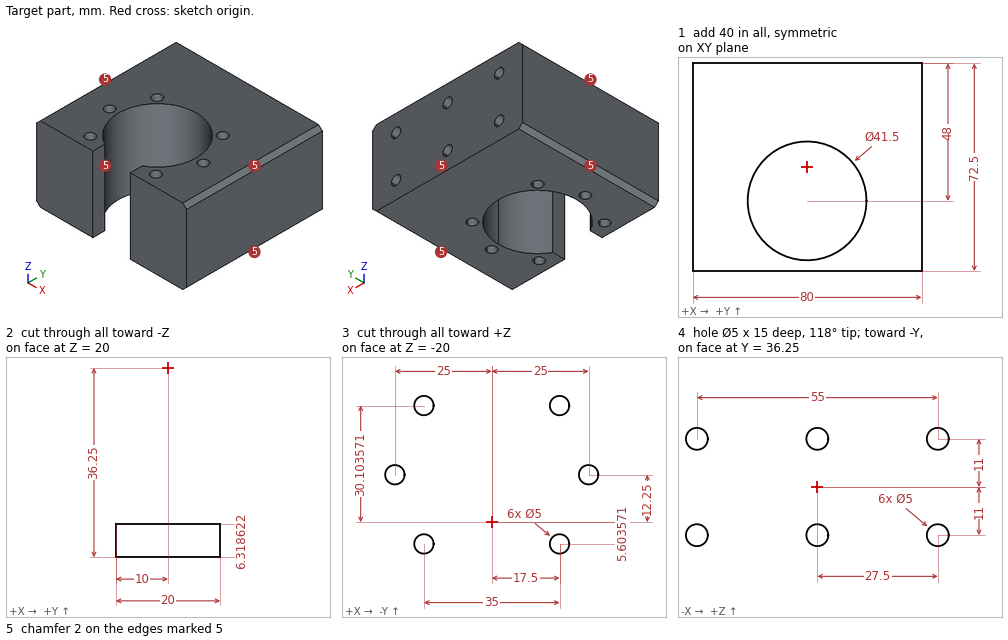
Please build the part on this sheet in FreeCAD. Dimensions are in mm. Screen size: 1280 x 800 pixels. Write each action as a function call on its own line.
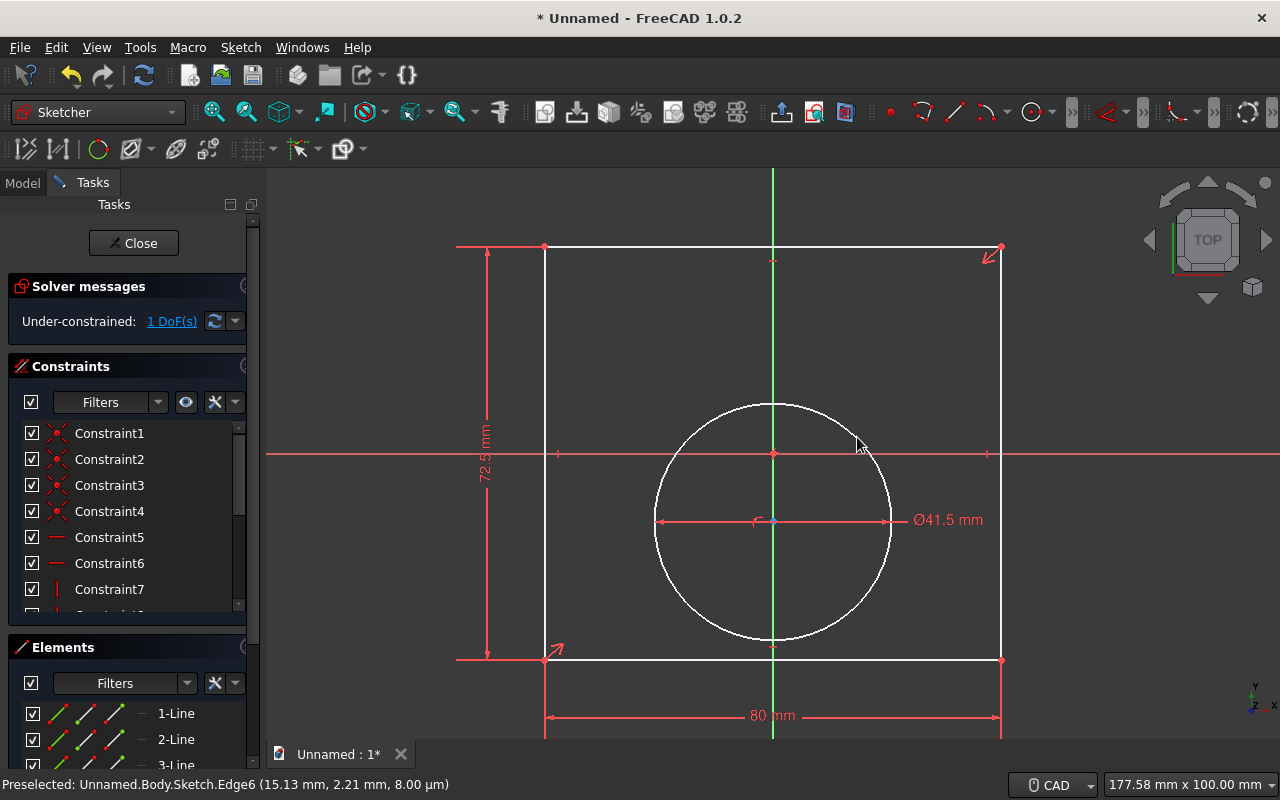
click(1106, 112)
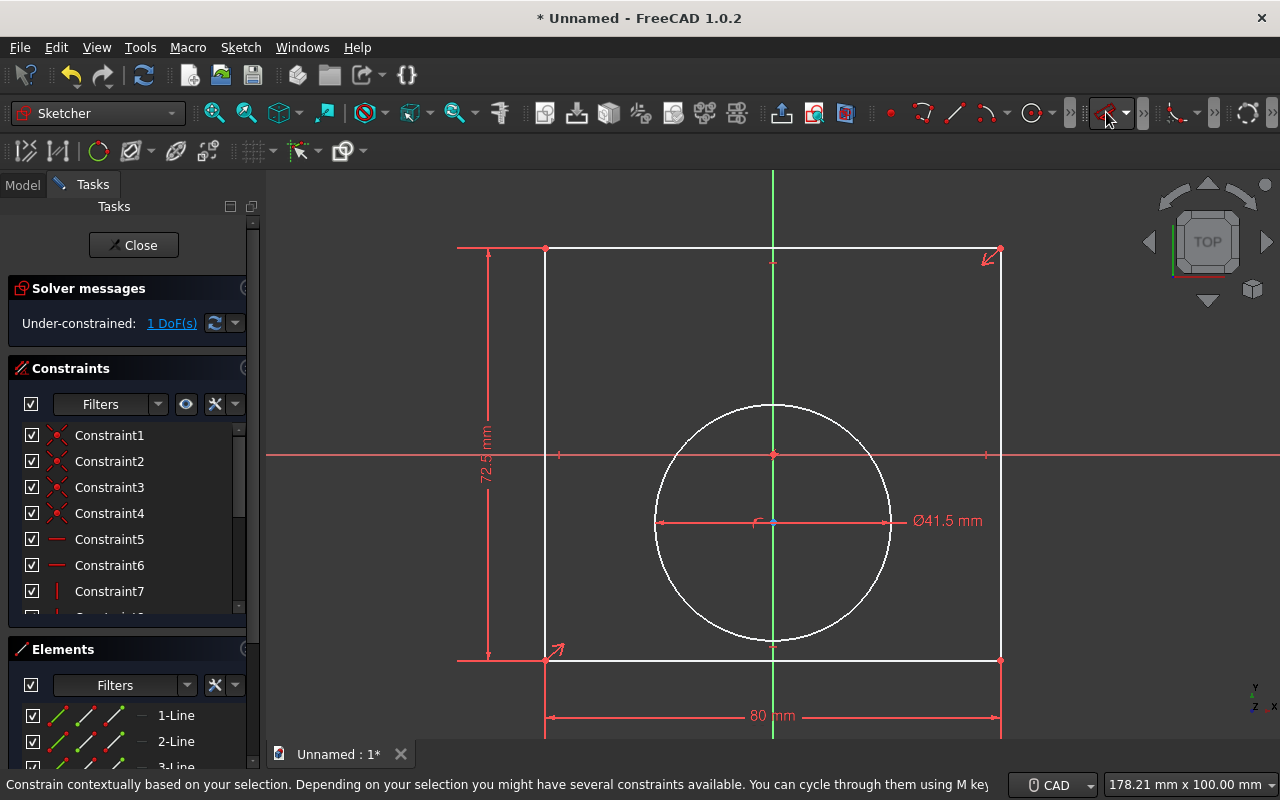
click(1001, 248)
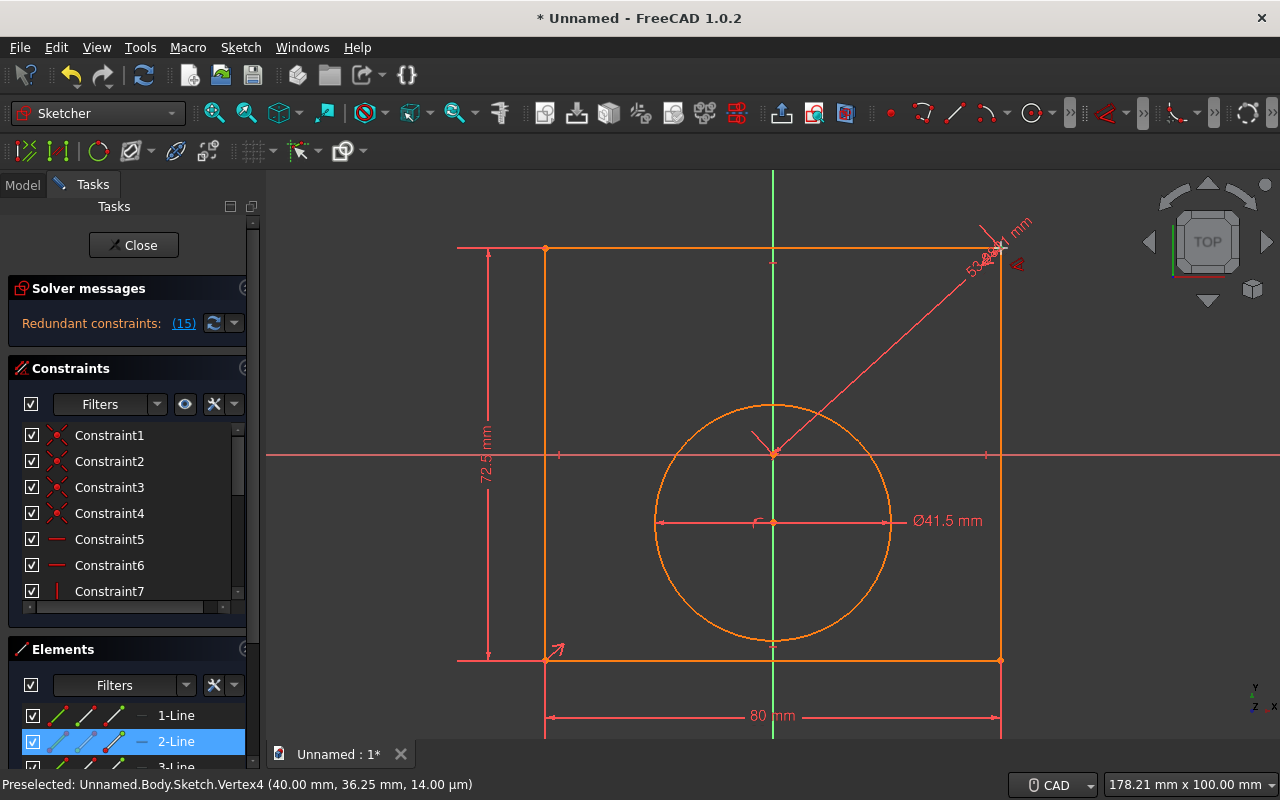
click(773, 523)
click(1035, 385)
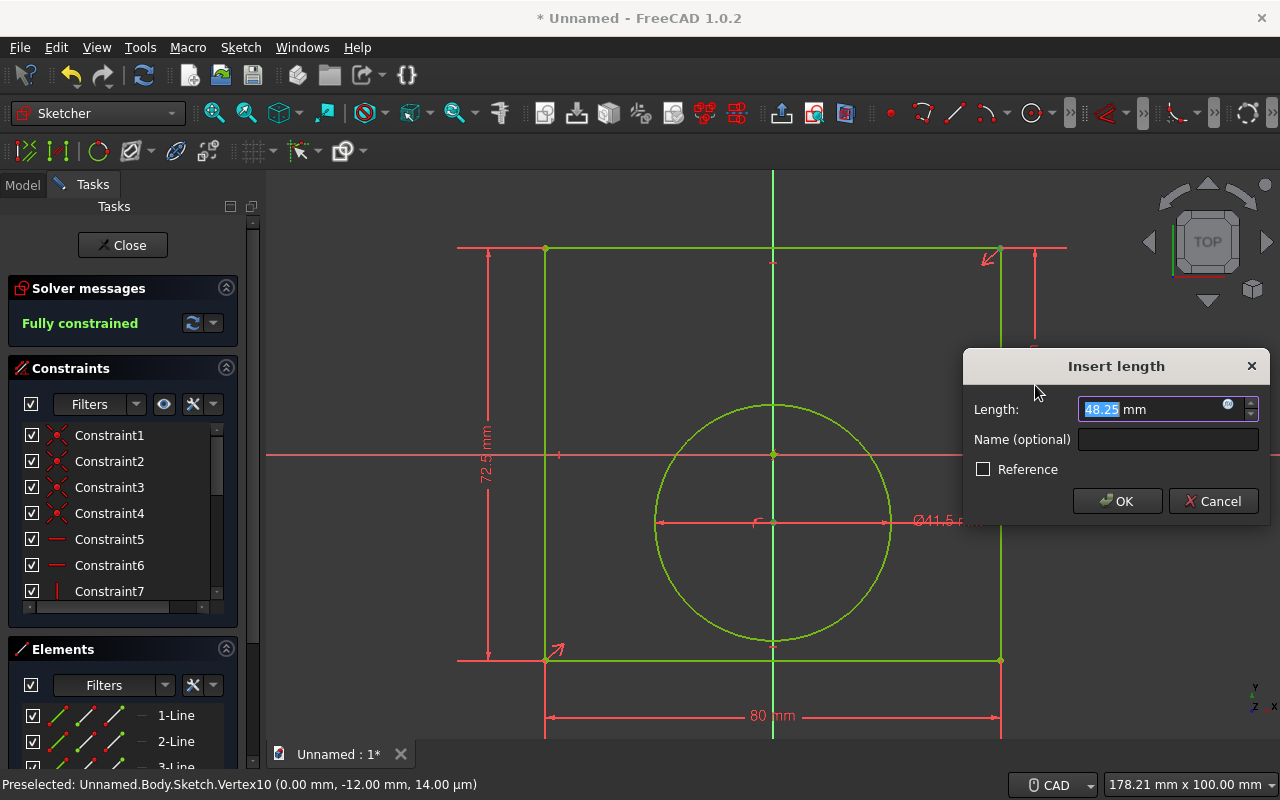
text(48)
key(Return)
key(Escape)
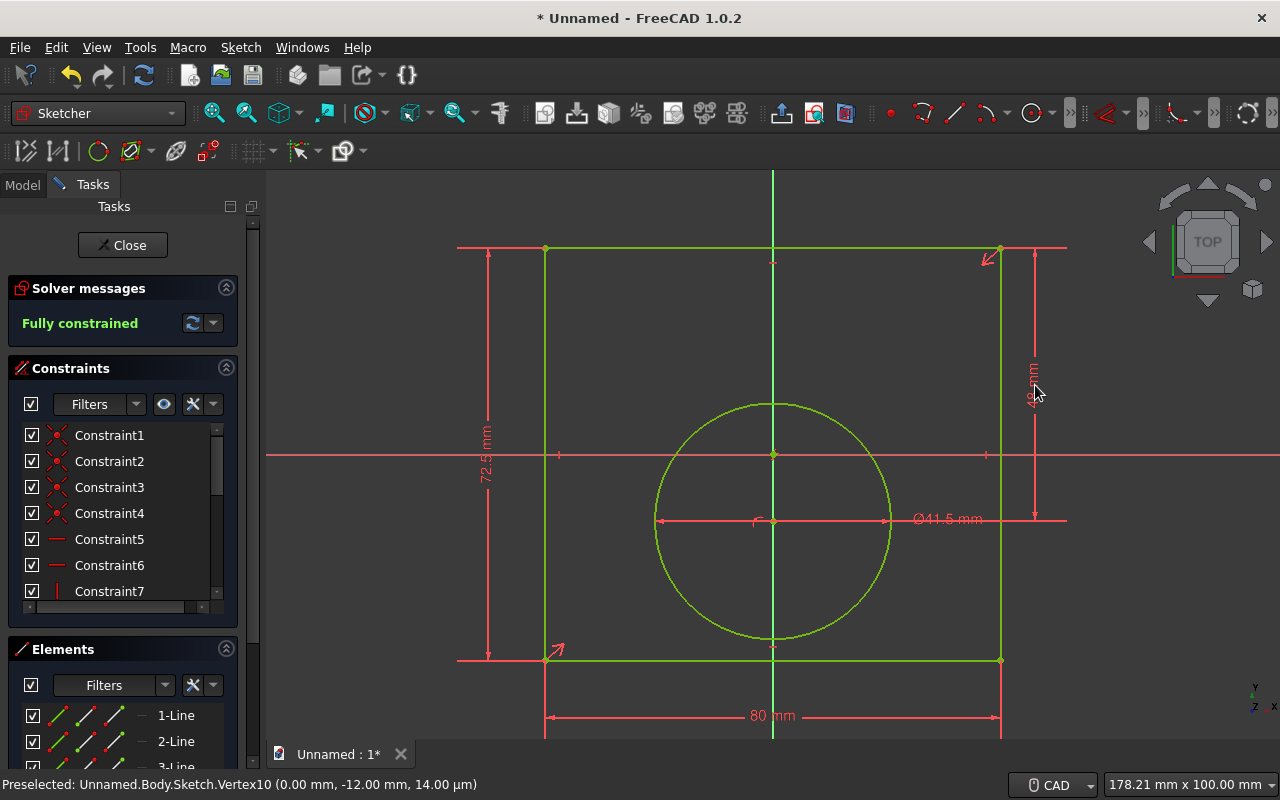
click(123, 245)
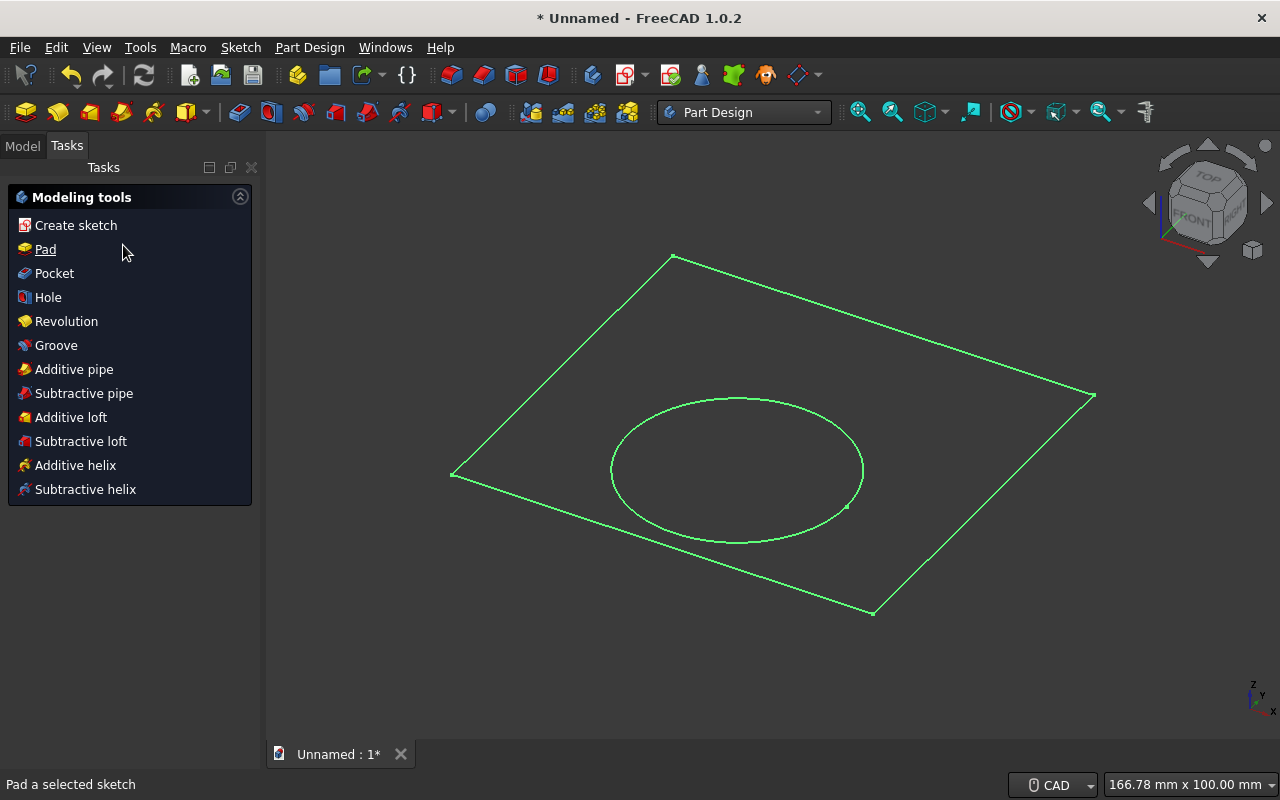
click(26, 112)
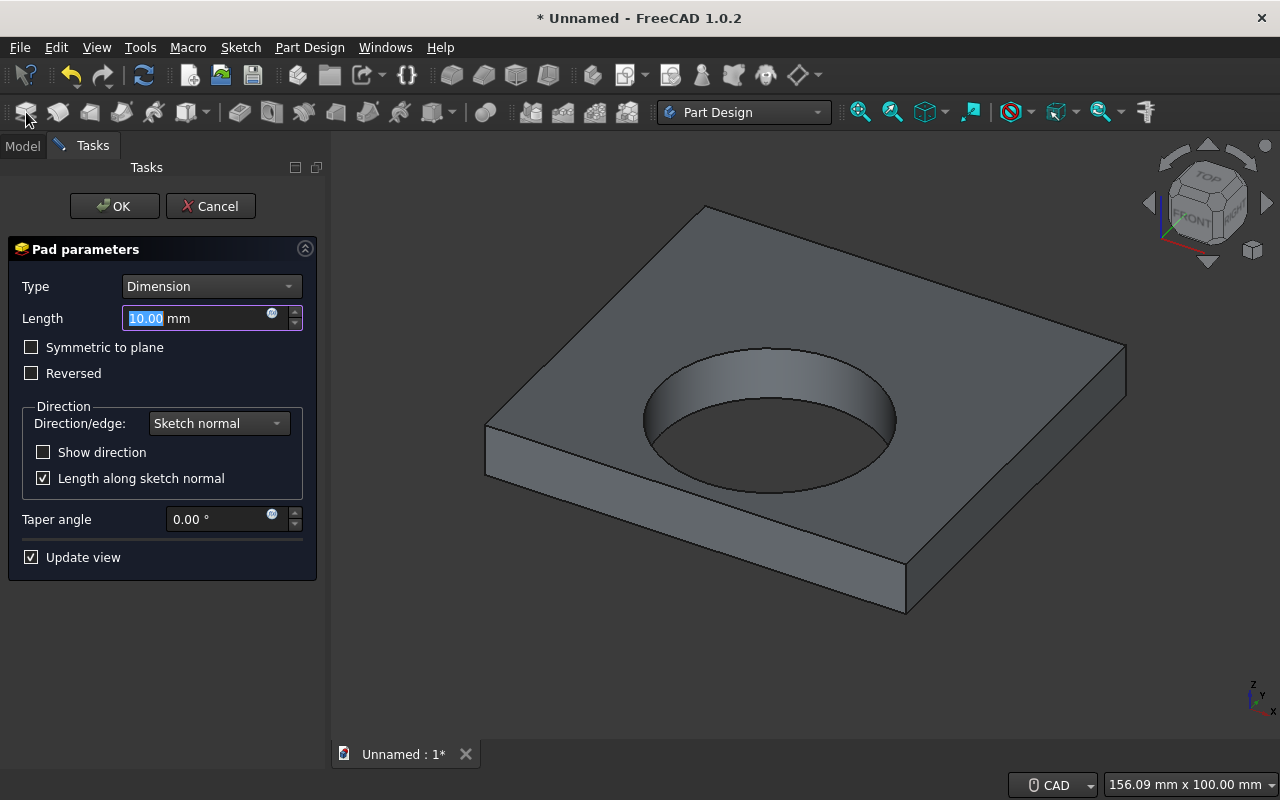
text(40)
key(Tab)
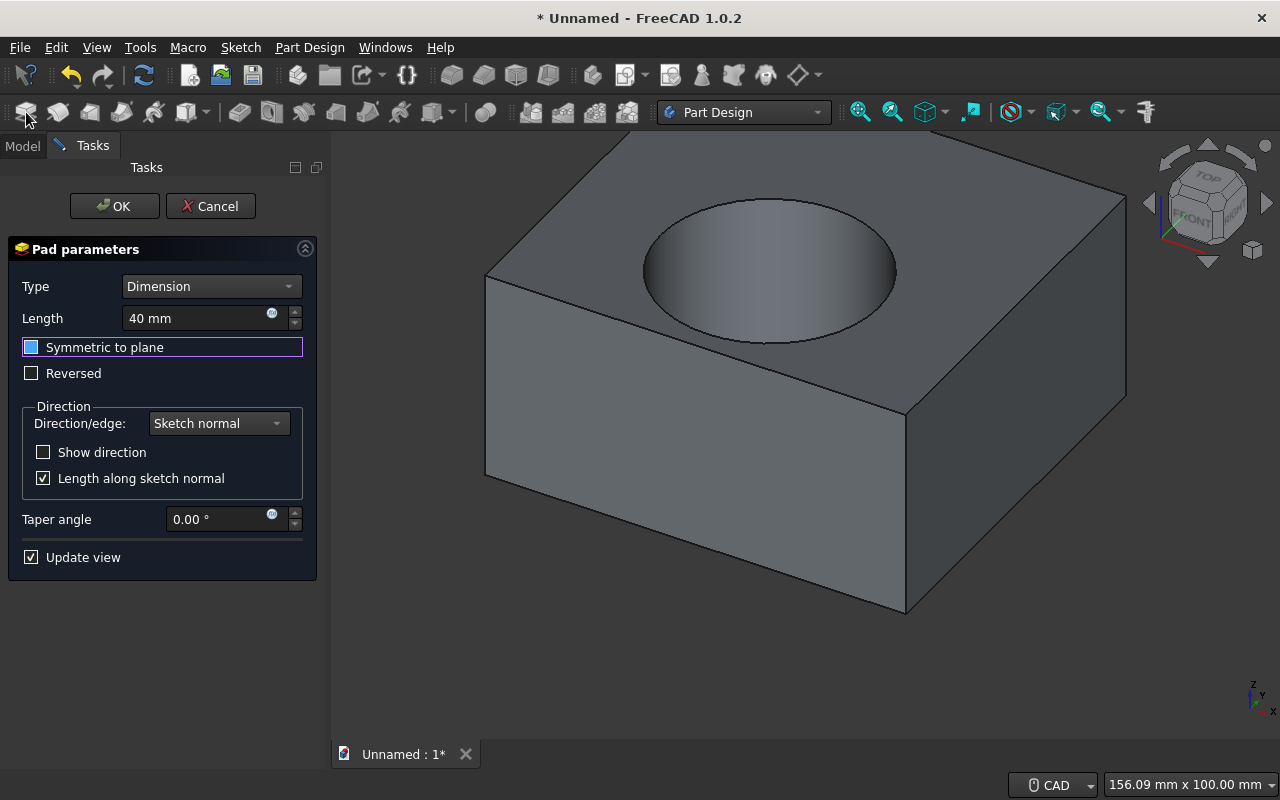
click(30, 347)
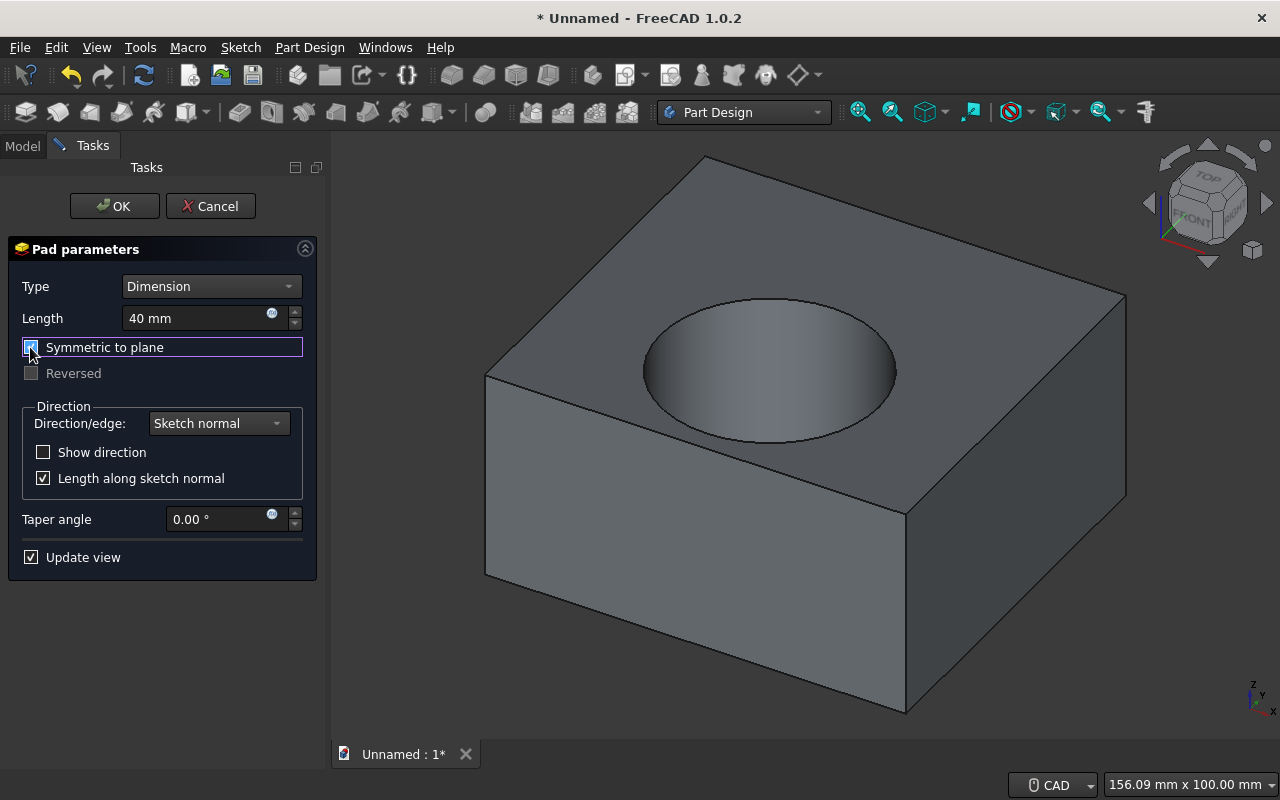
click(115, 206)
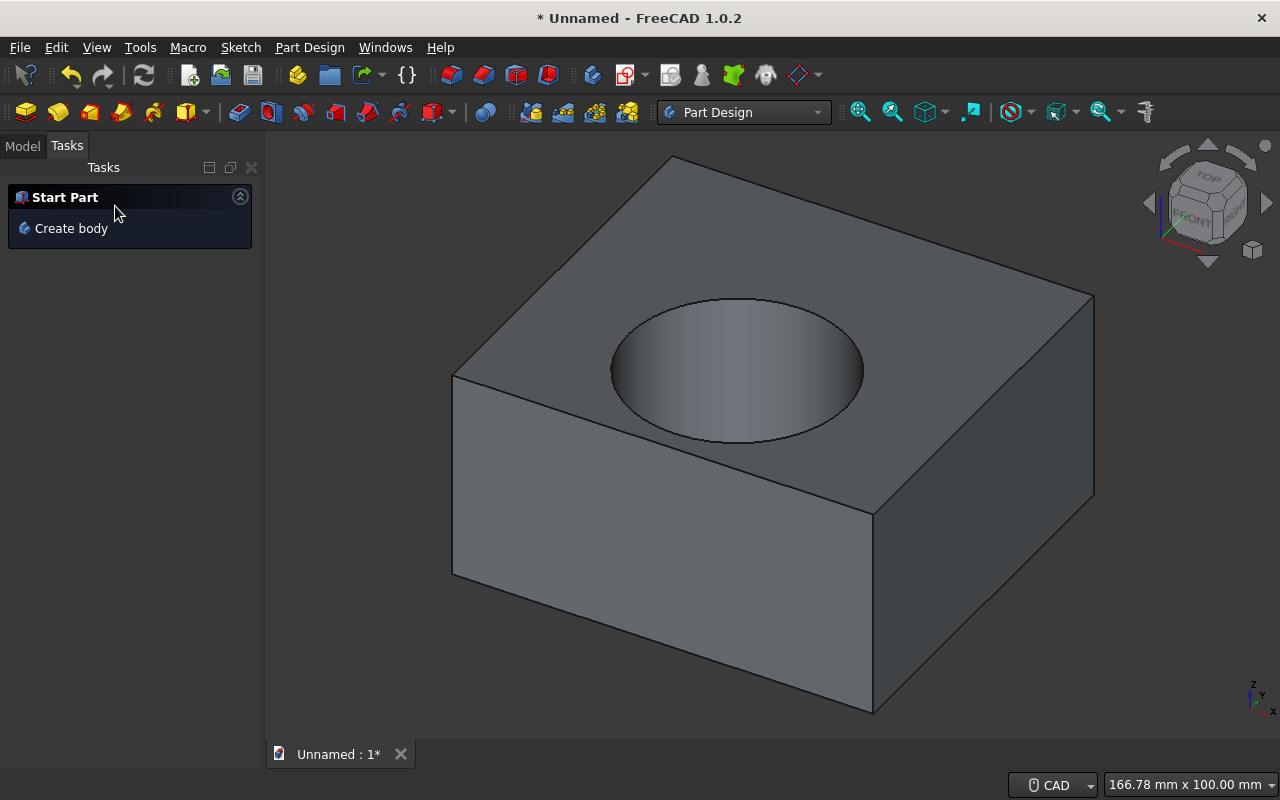
click(956, 312)